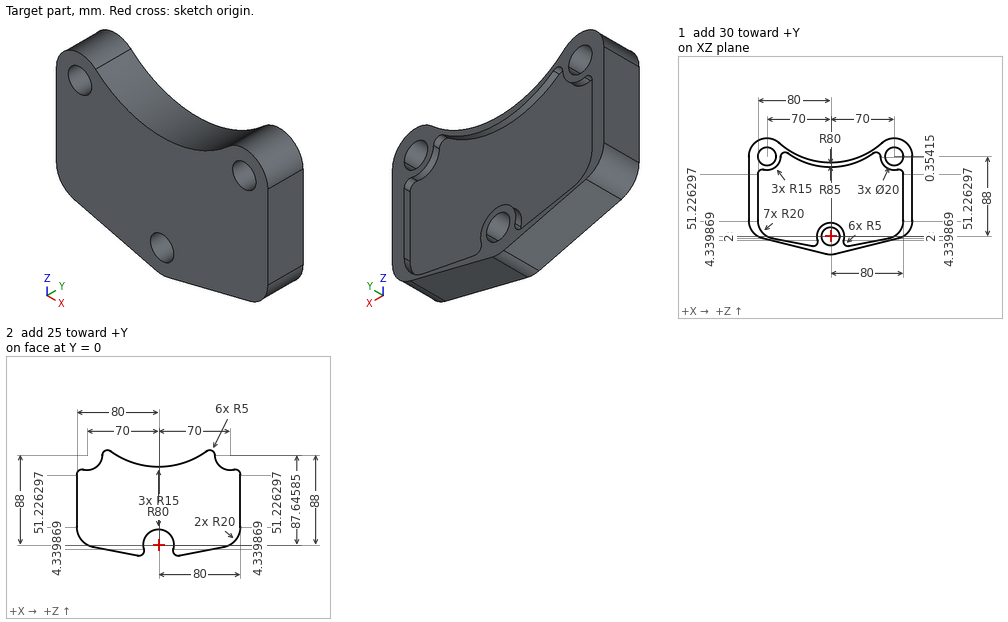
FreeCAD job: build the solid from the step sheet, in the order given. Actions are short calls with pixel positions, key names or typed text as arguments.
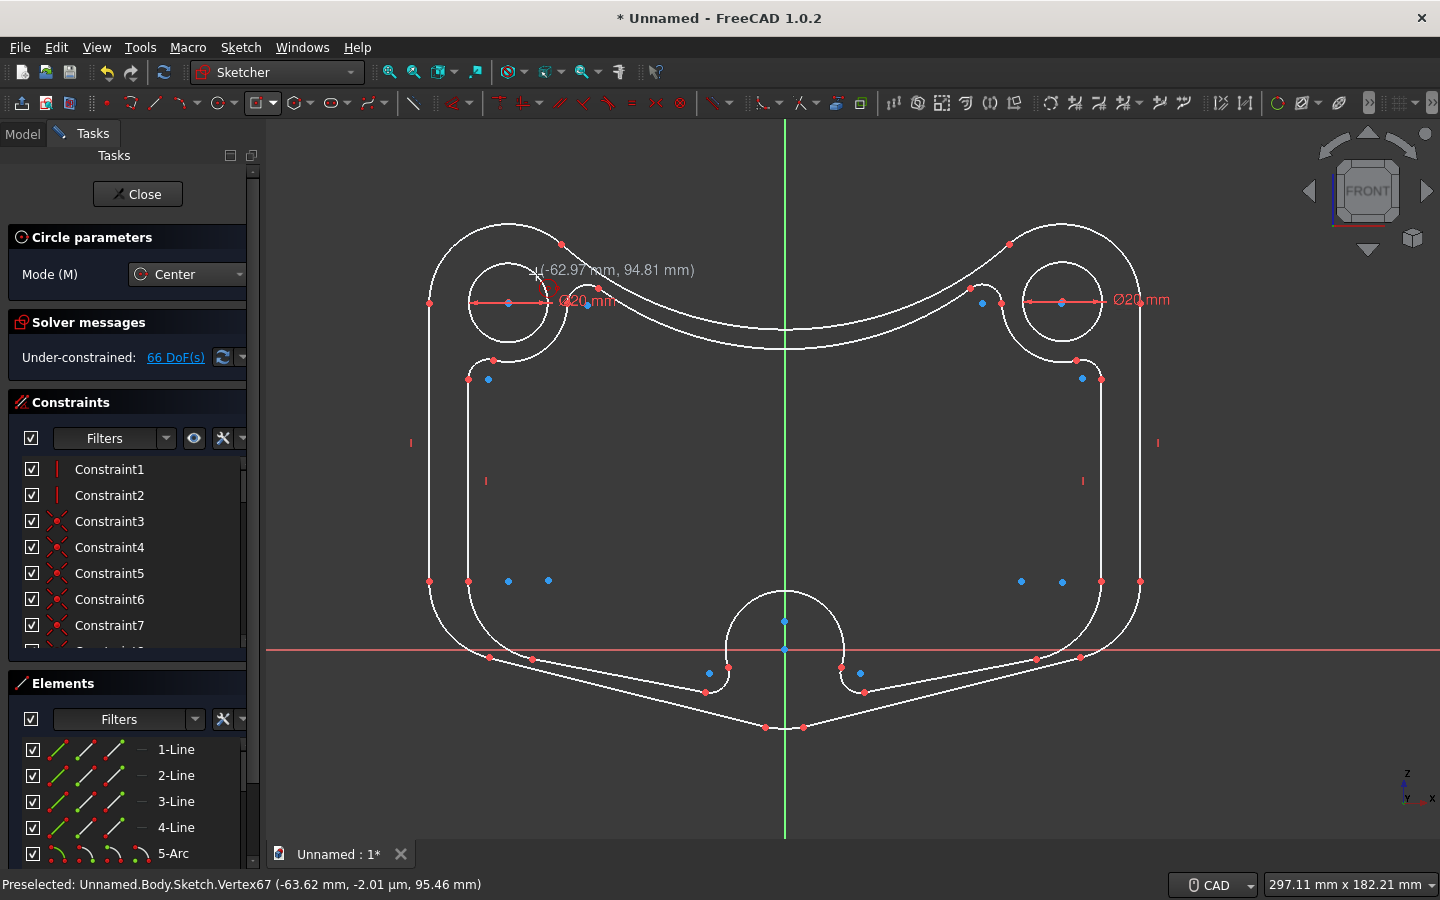
click(785, 650)
move(813, 622)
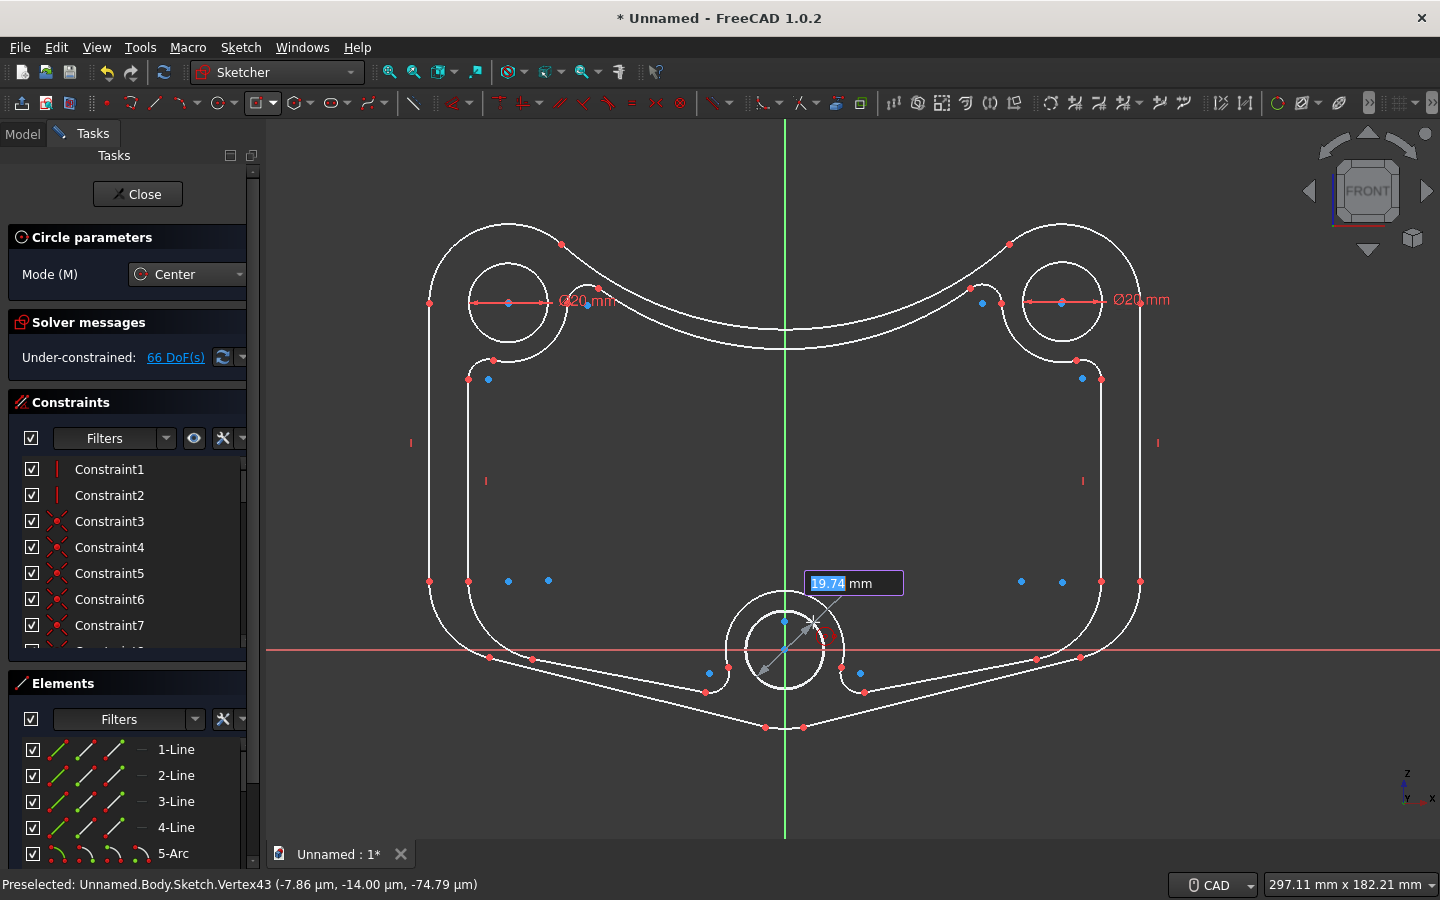
text(20)
key(Return)
key(Escape)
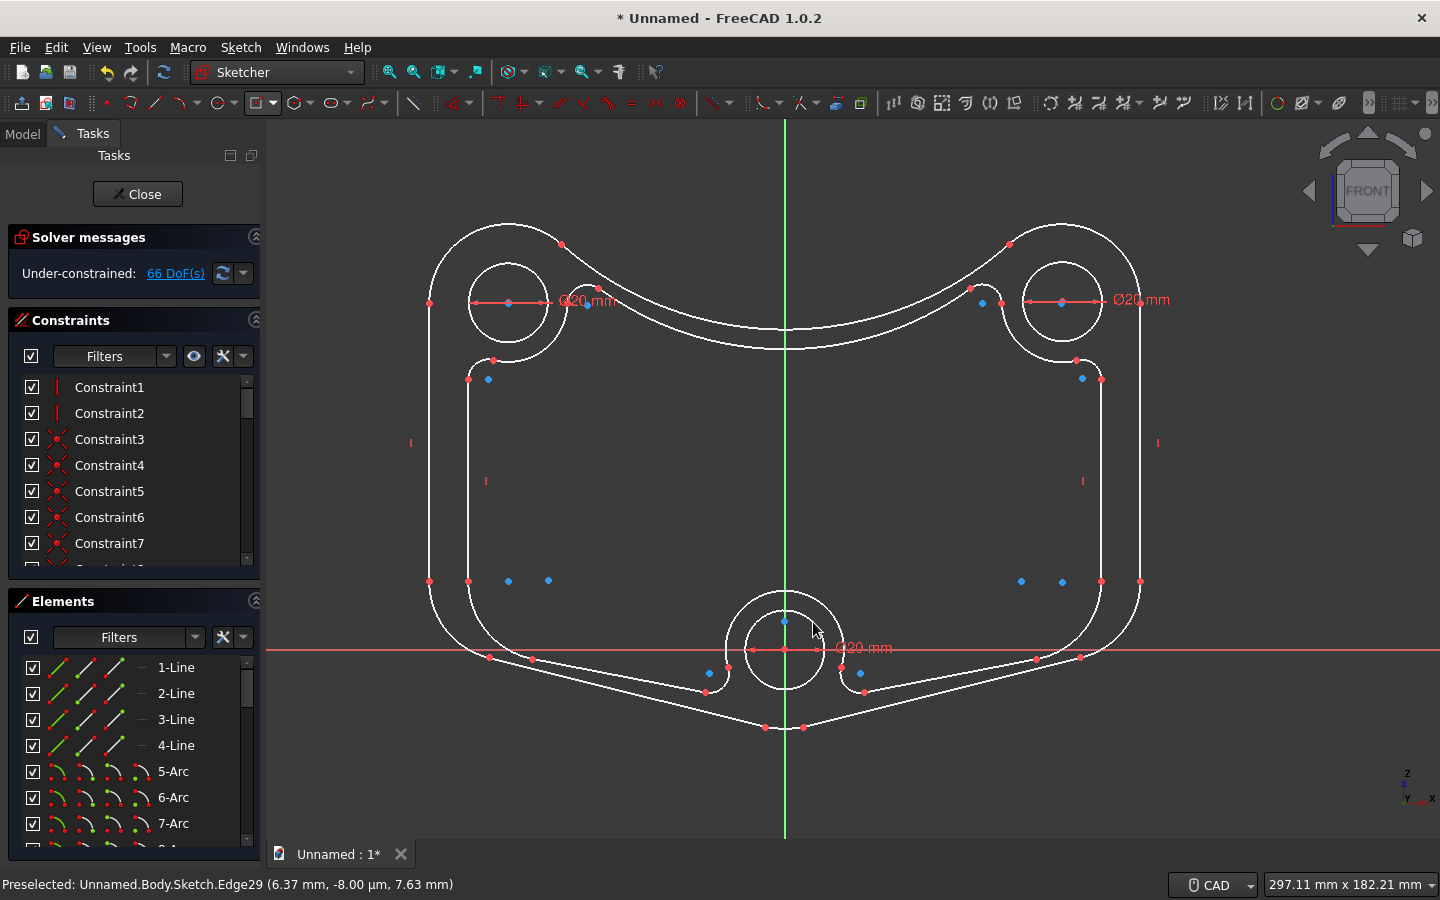
click(429, 498)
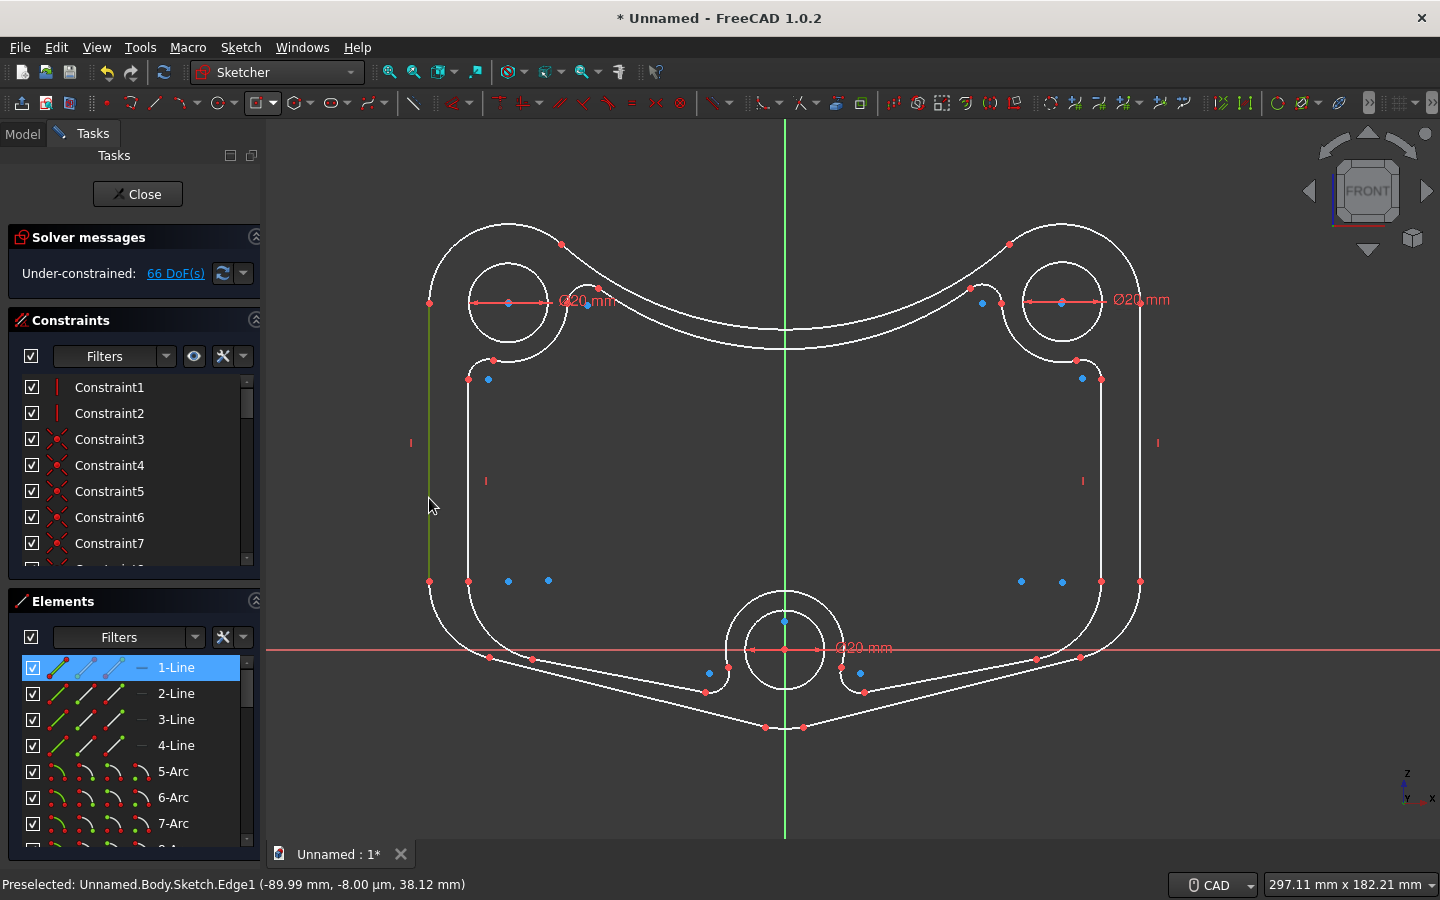
click(511, 224)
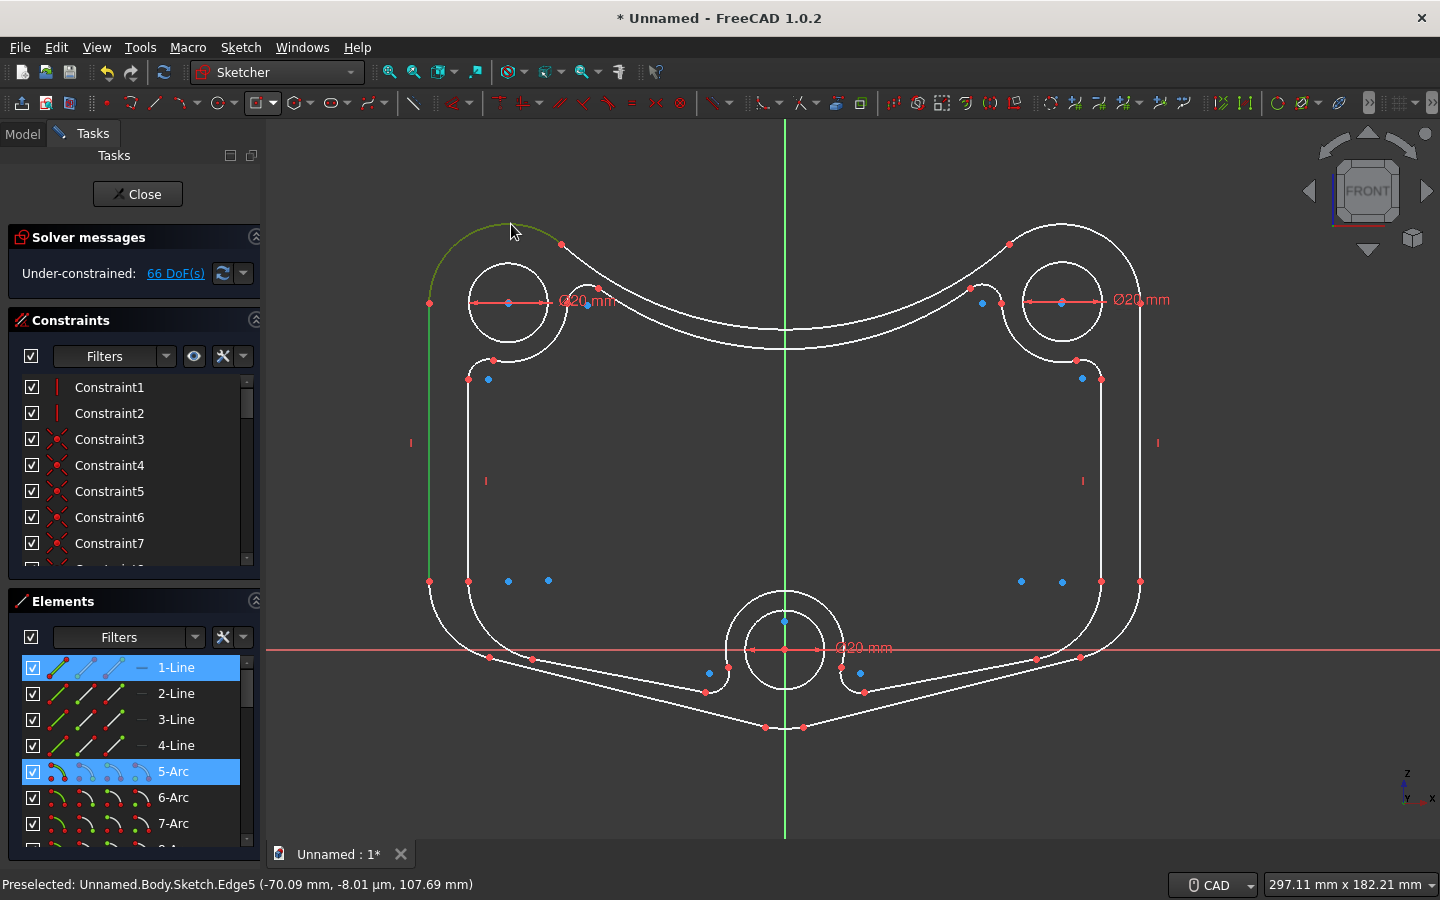
click(608, 104)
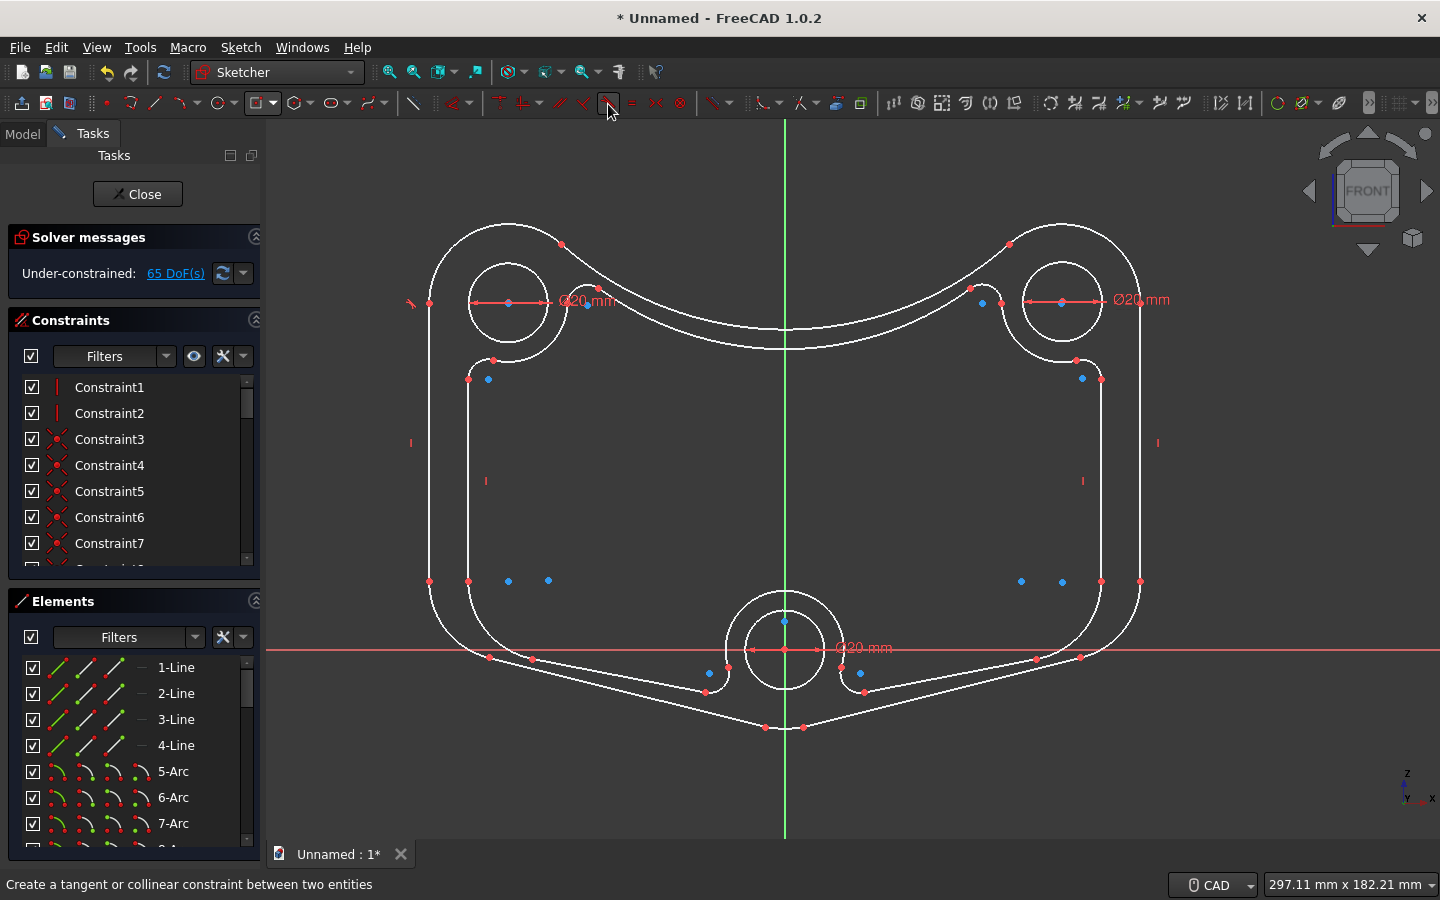
click(429, 498)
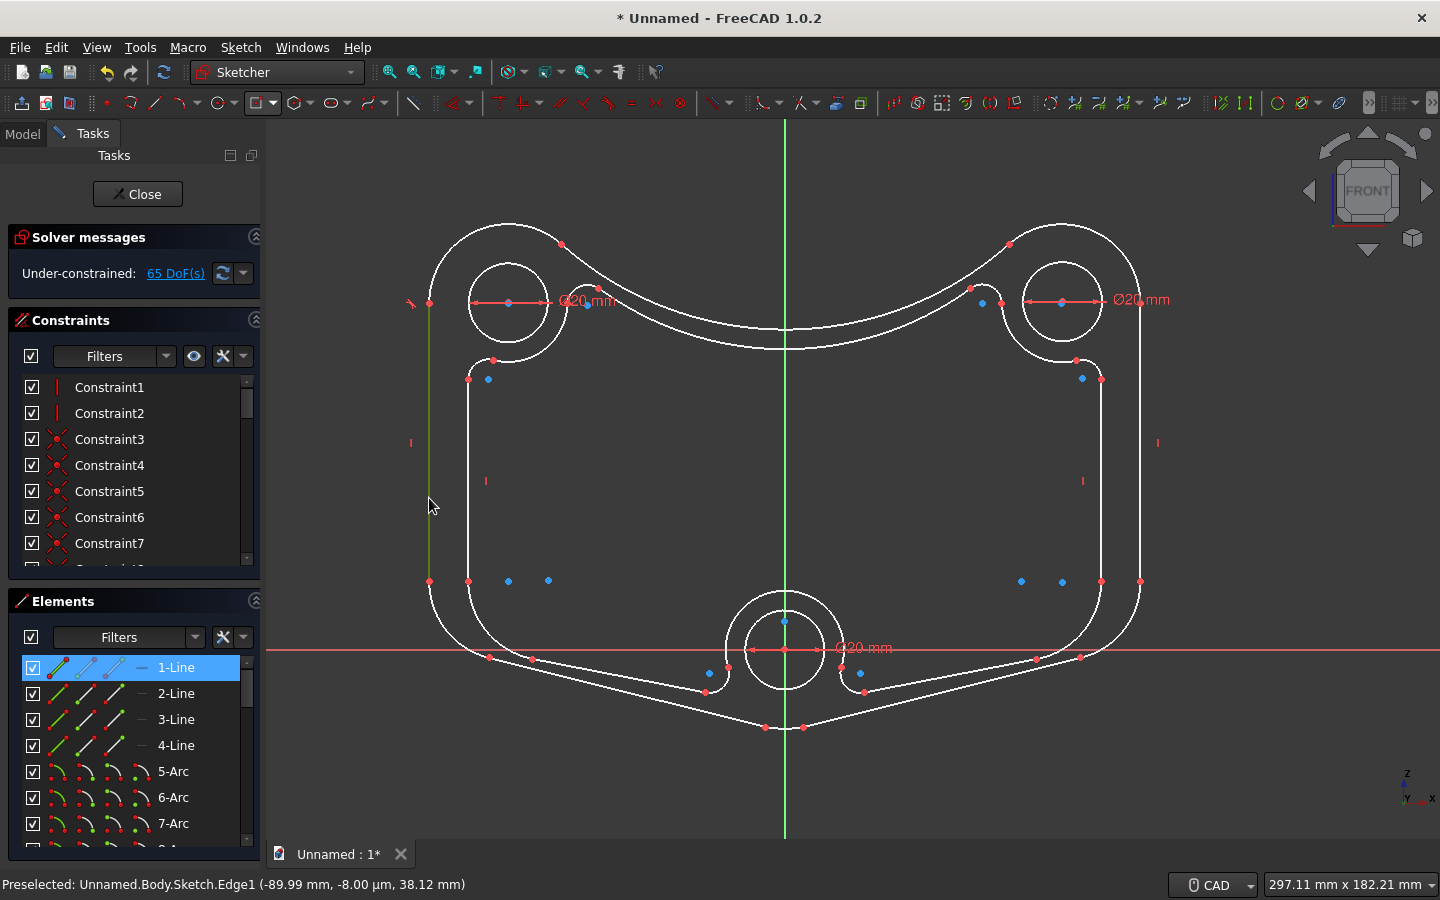
click(435, 612)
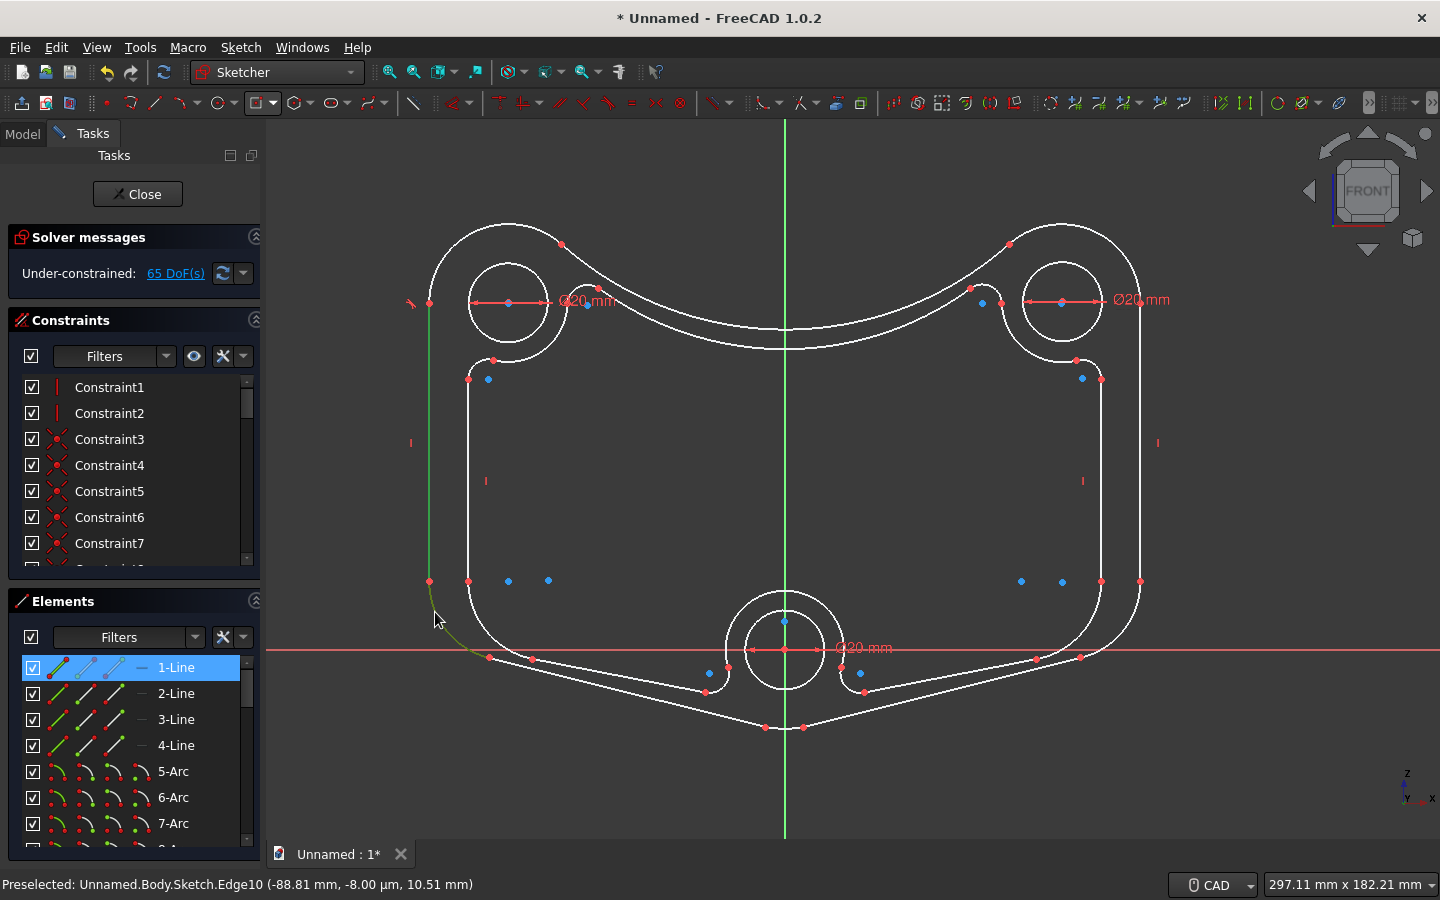
click(608, 104)